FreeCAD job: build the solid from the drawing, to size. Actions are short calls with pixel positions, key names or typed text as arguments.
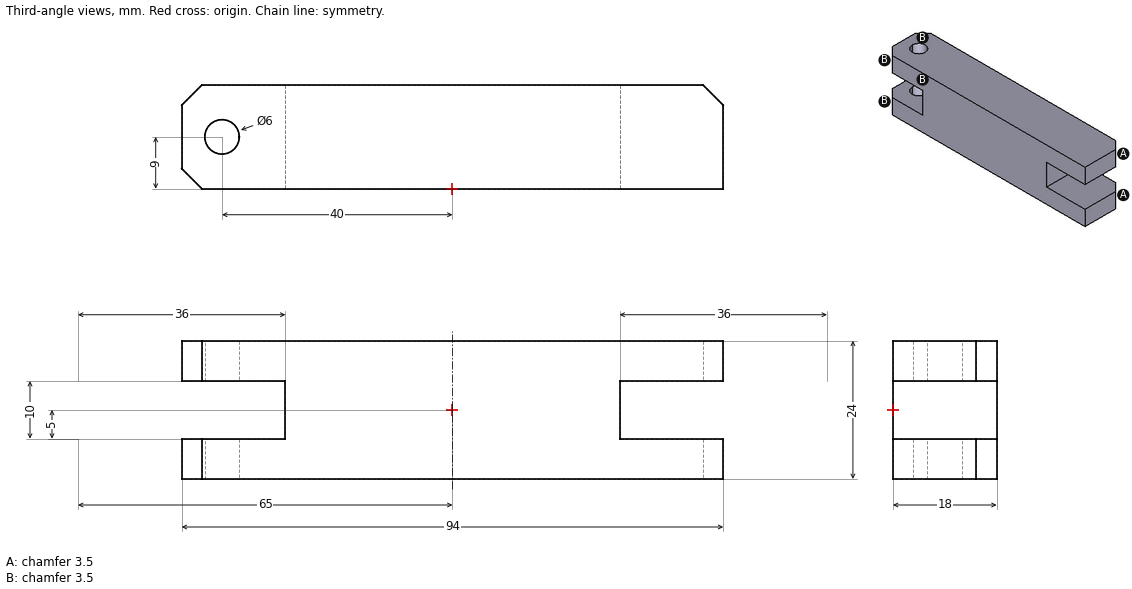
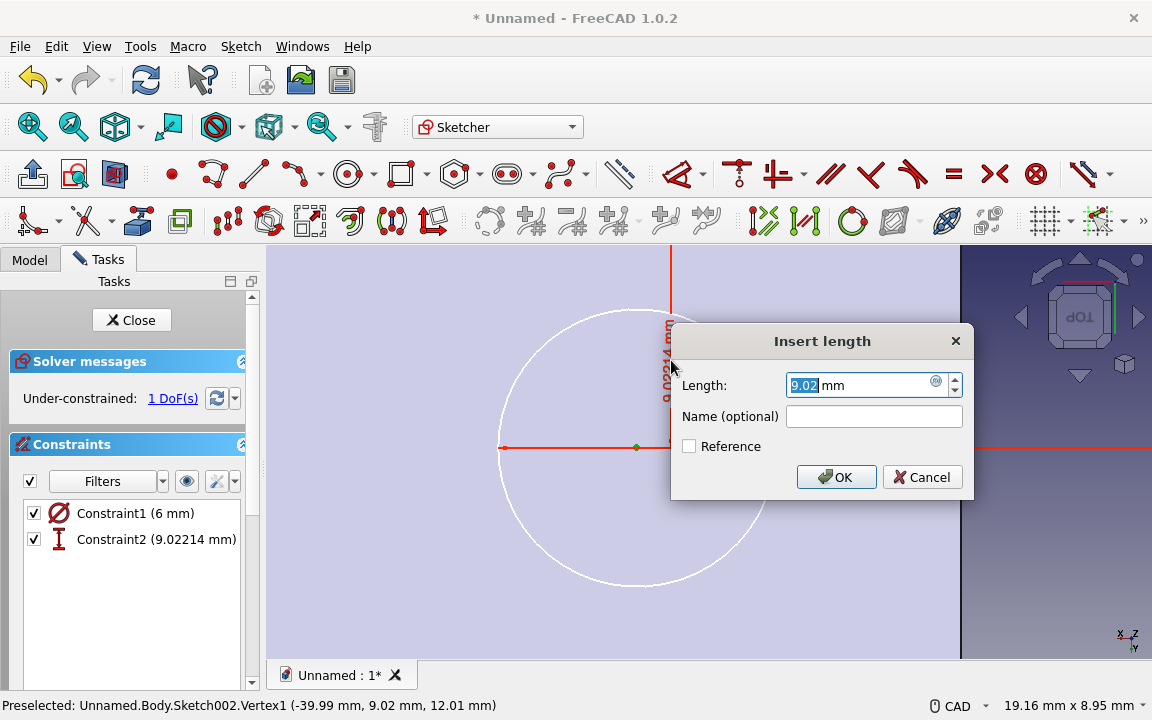
text(9)
key(Return)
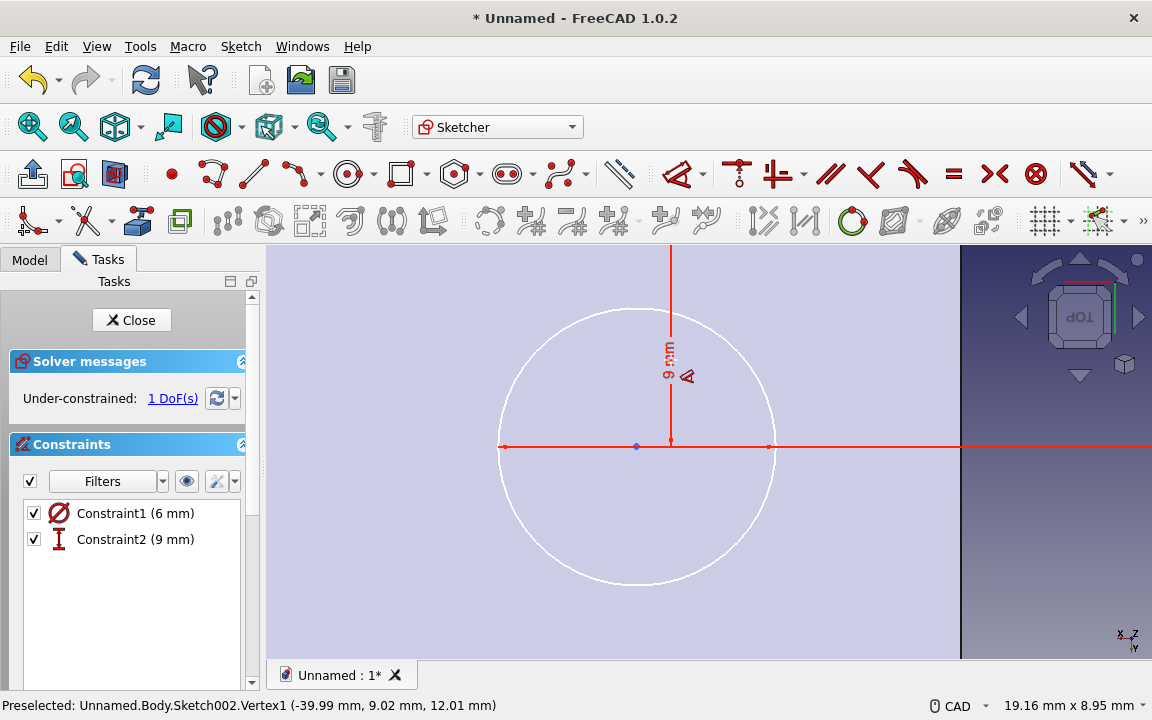
click(637, 447)
click(465, 481)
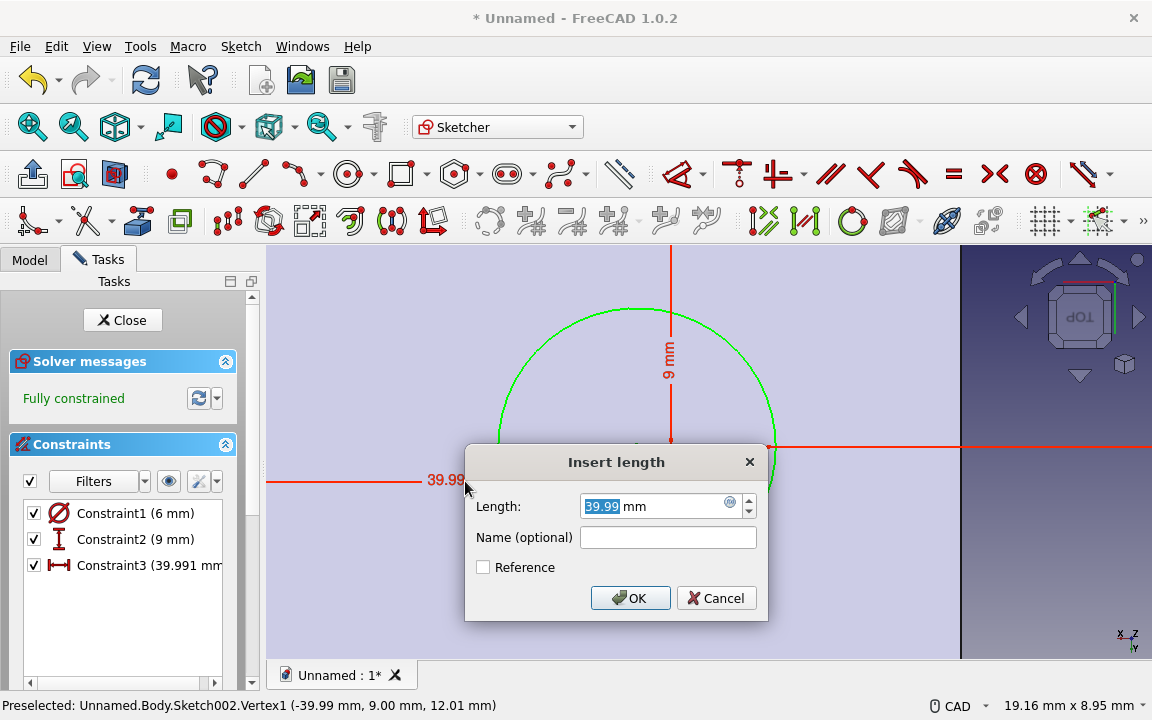
text(40)
key(Return)
key(Escape)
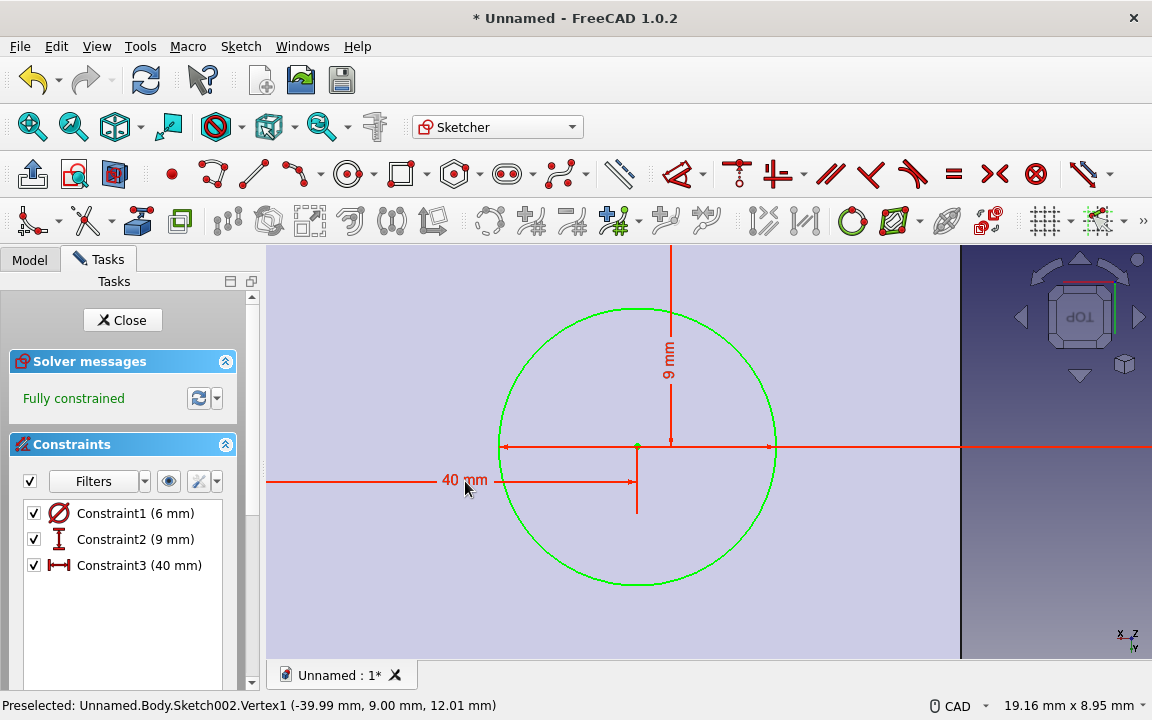
click(123, 320)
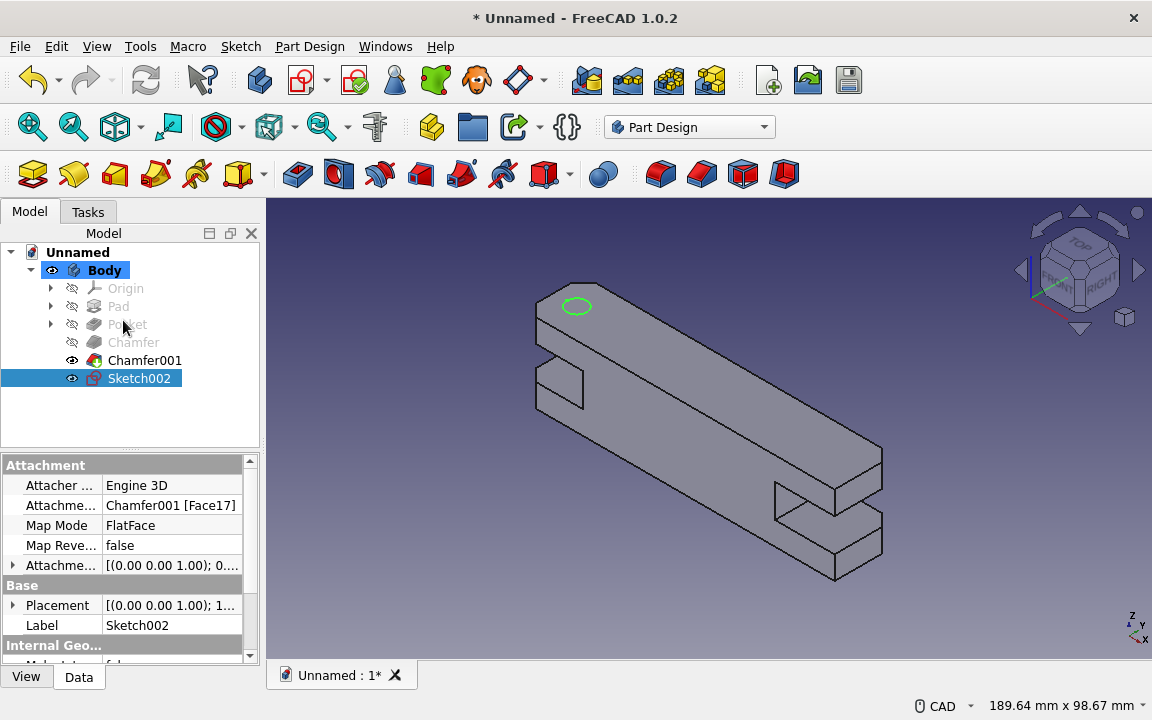
click(298, 174)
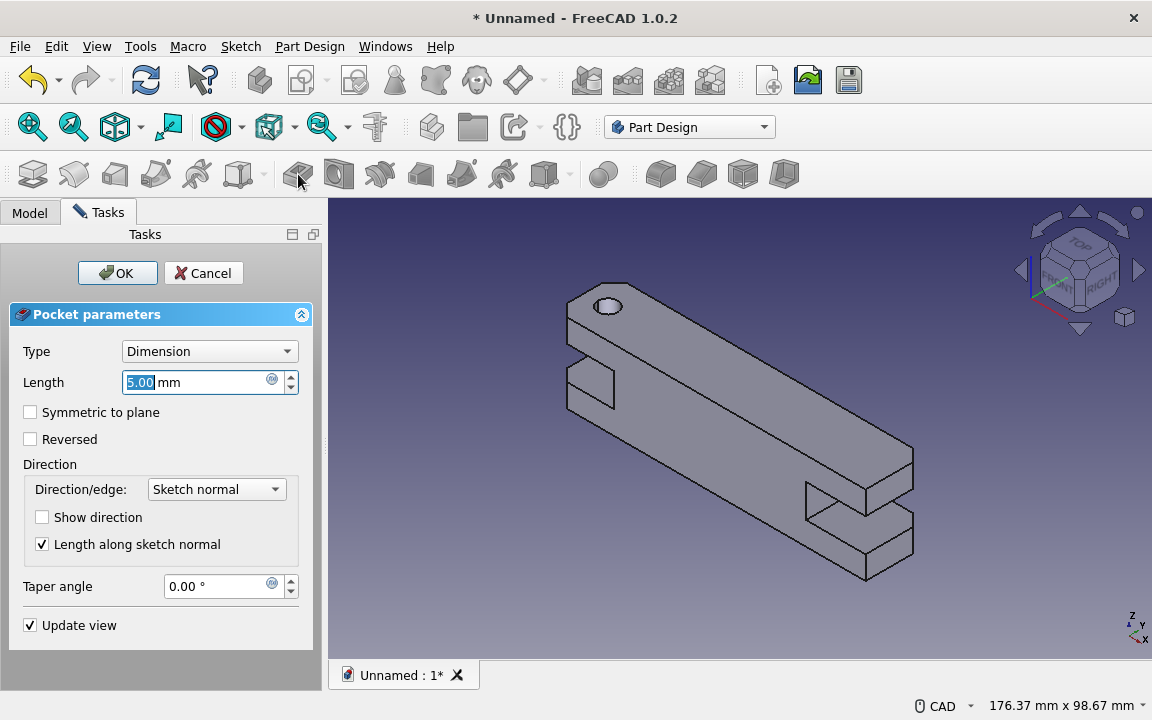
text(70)
key(Tab)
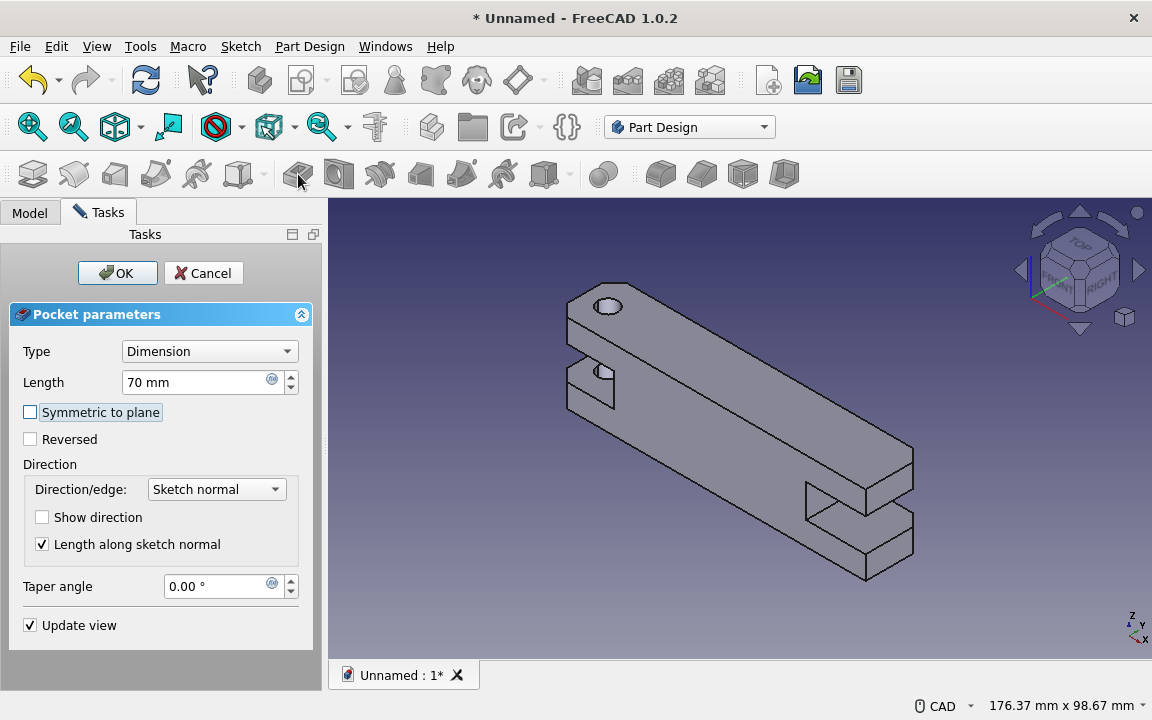
click(118, 273)